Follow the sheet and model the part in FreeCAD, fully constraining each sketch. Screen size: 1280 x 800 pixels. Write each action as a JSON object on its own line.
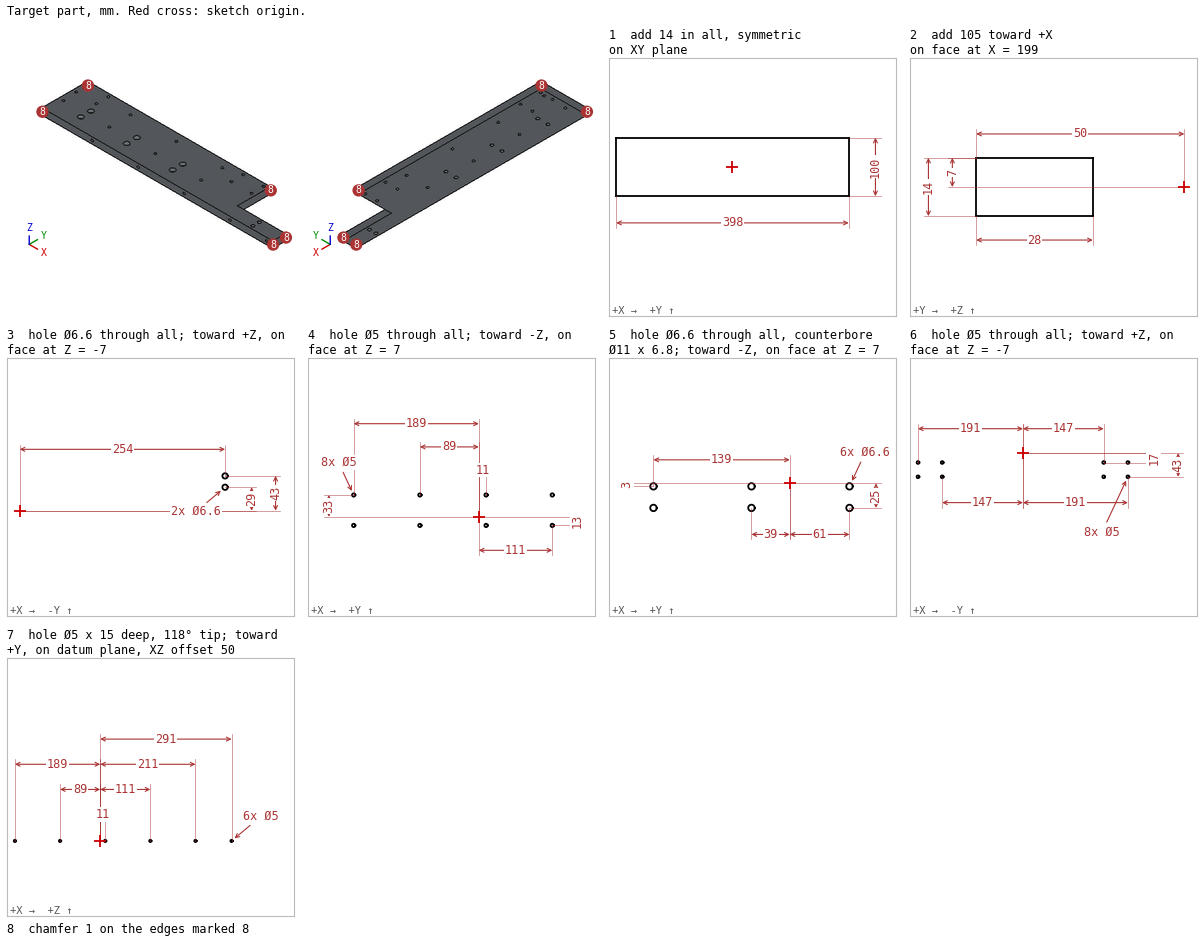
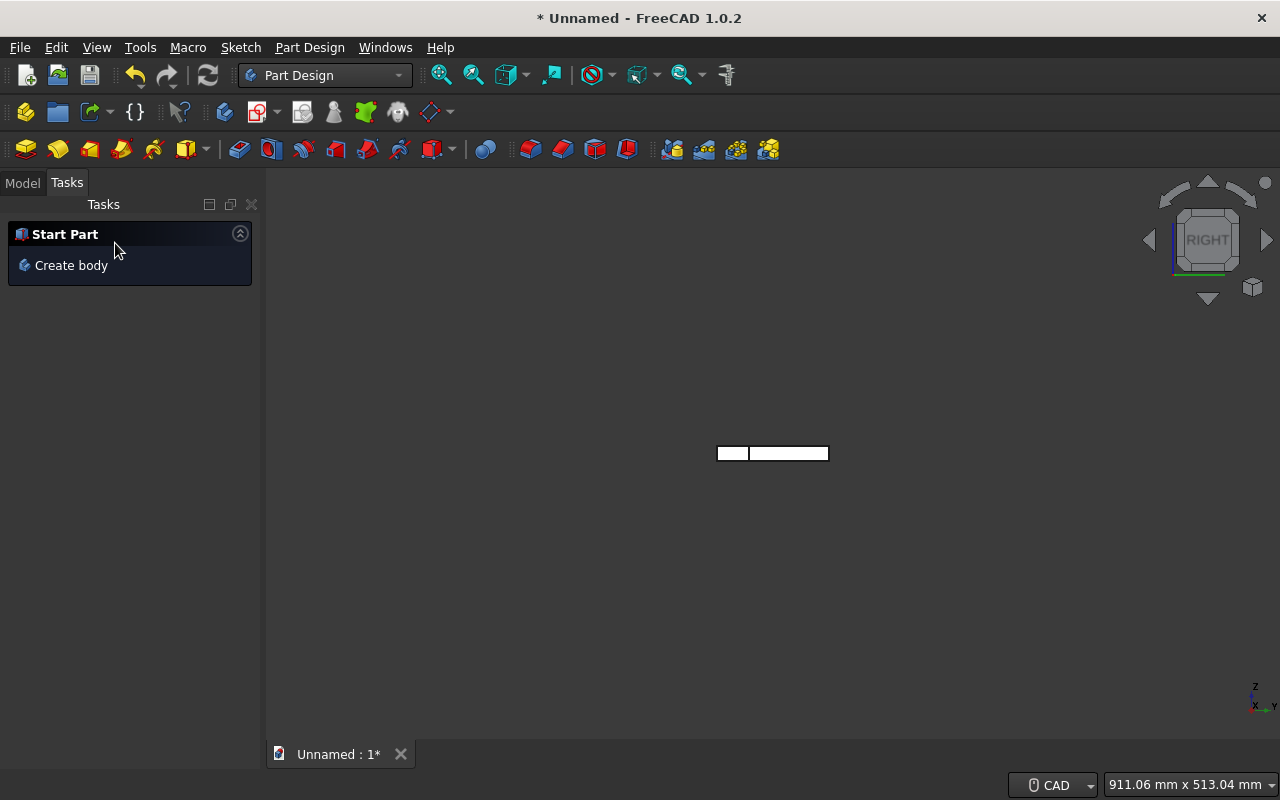
{"action": "key", "text": "5"}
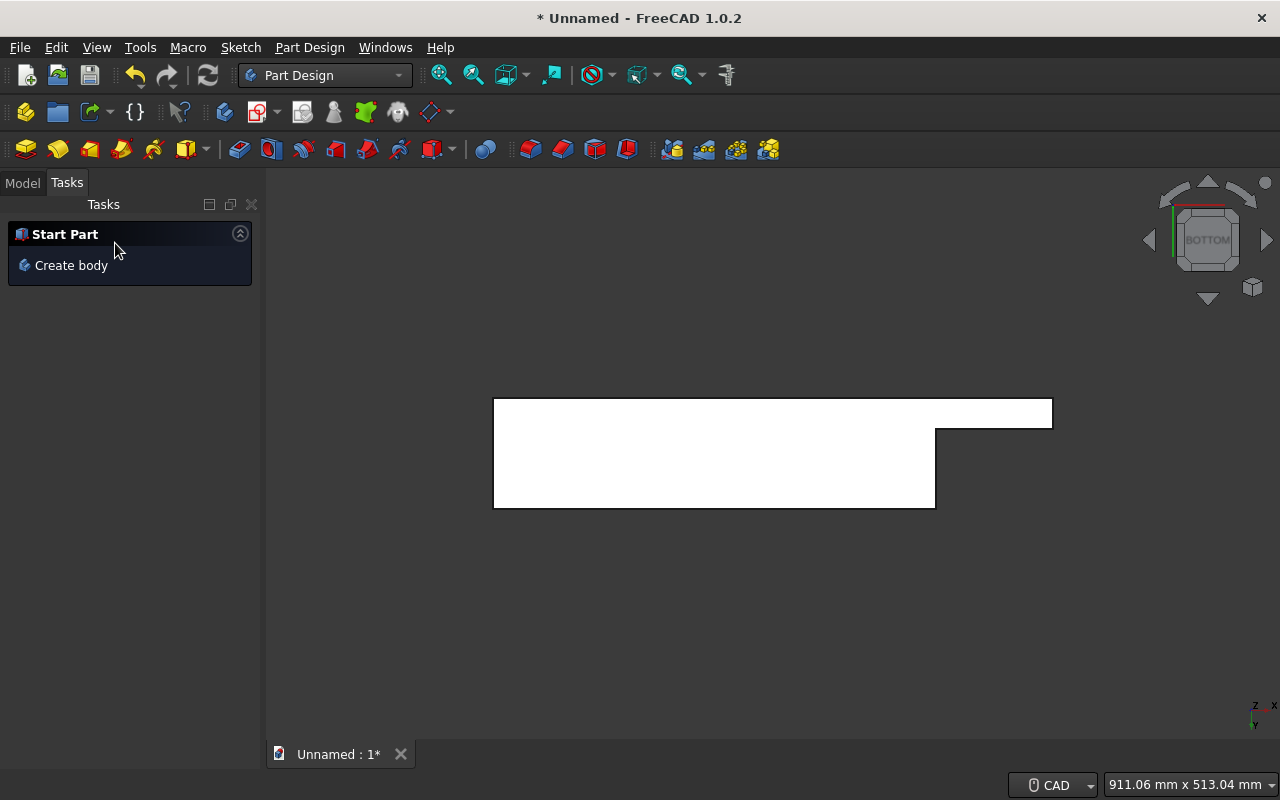
{"action": "left_click", "coordinate": [853, 452]}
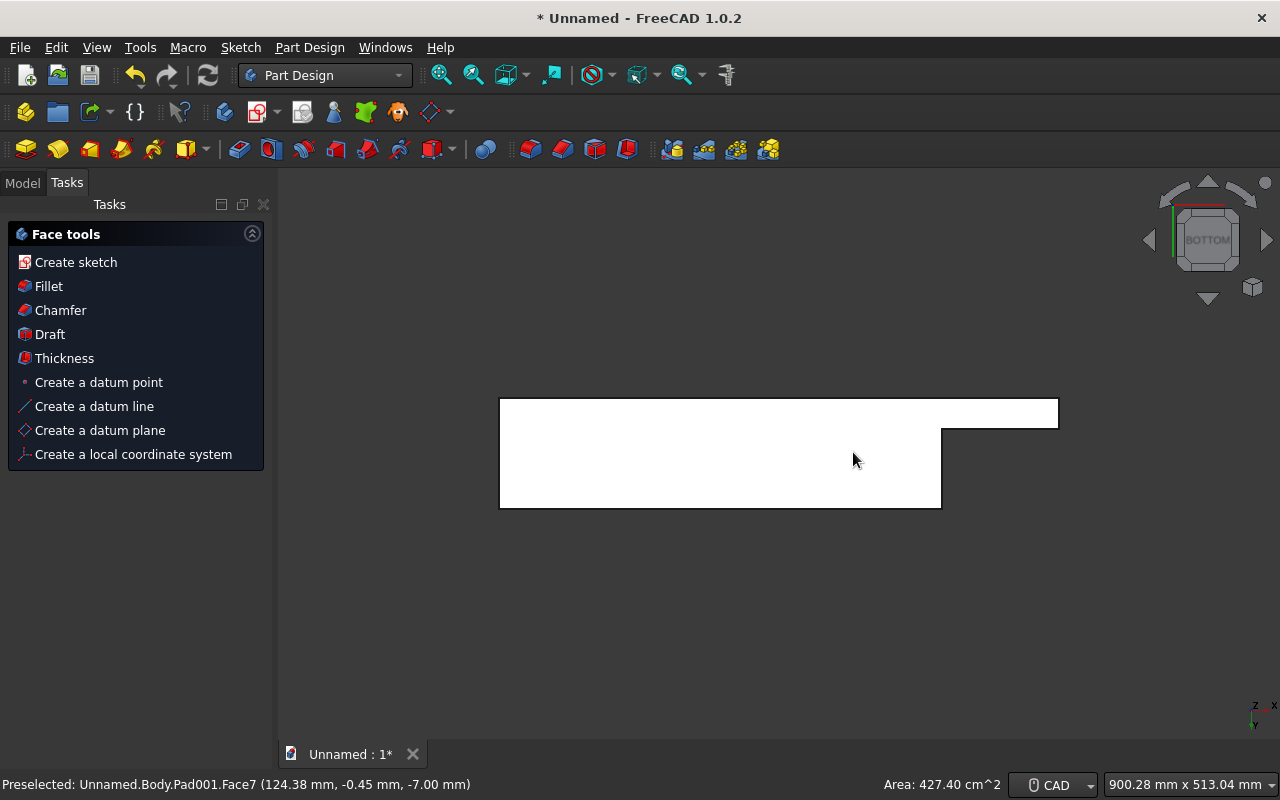
{"action": "left_click", "coordinate": [258, 112]}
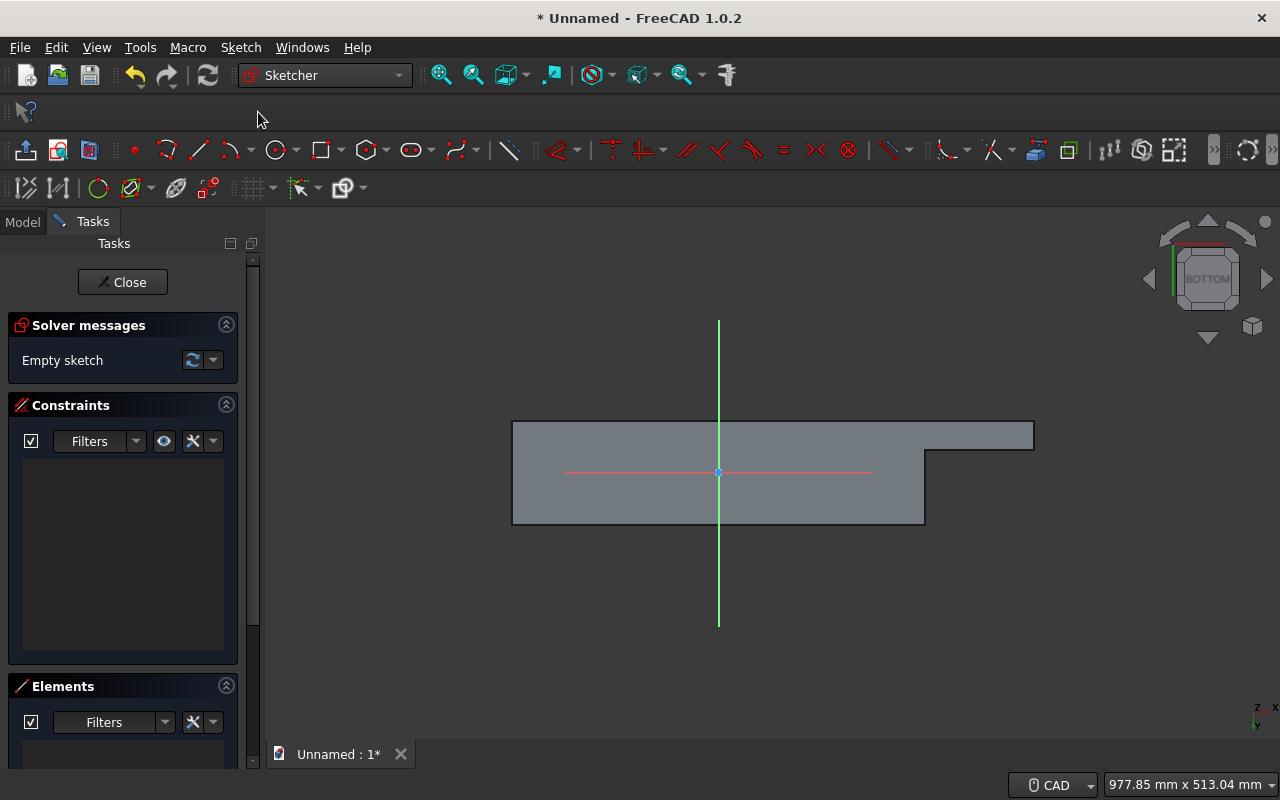
{"action": "scroll", "coordinate": [1000, 433], "scroll_direction": "up", "scroll_amount": 14}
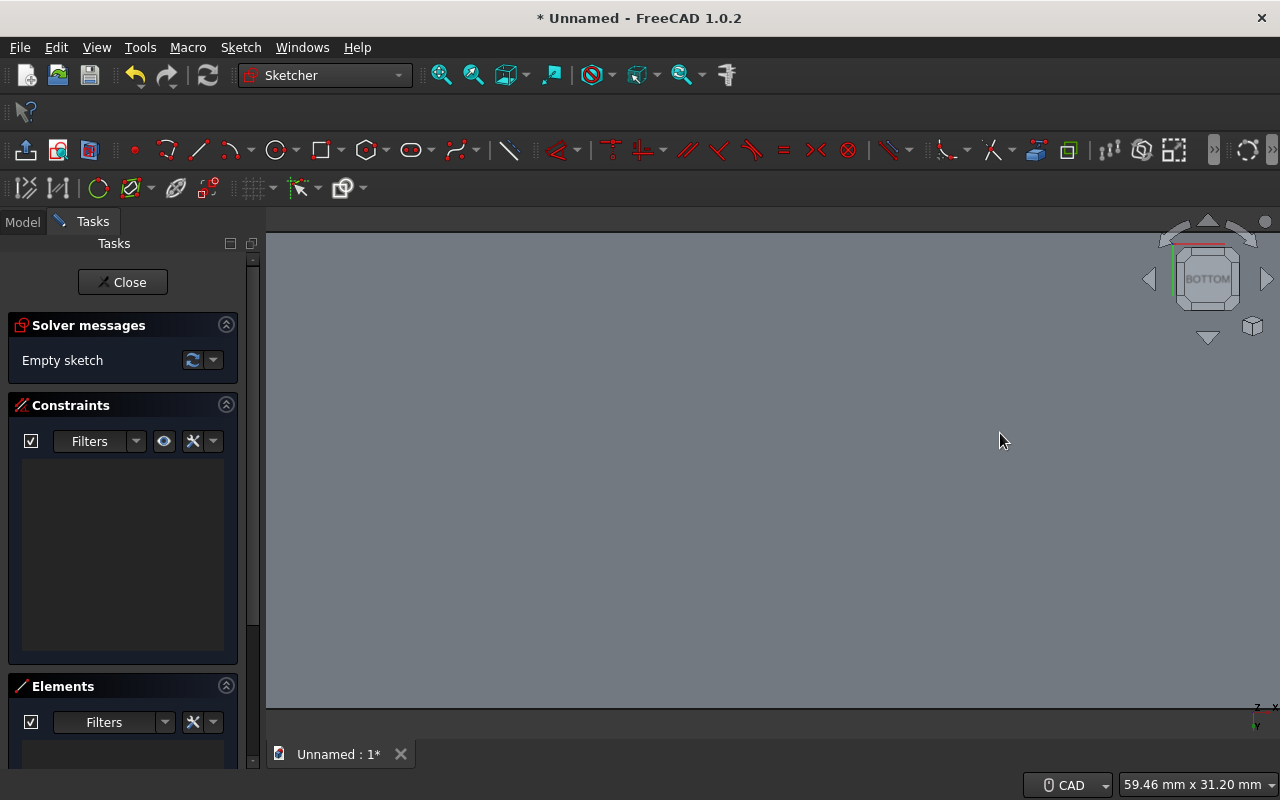
{"action": "key", "text": "g c"}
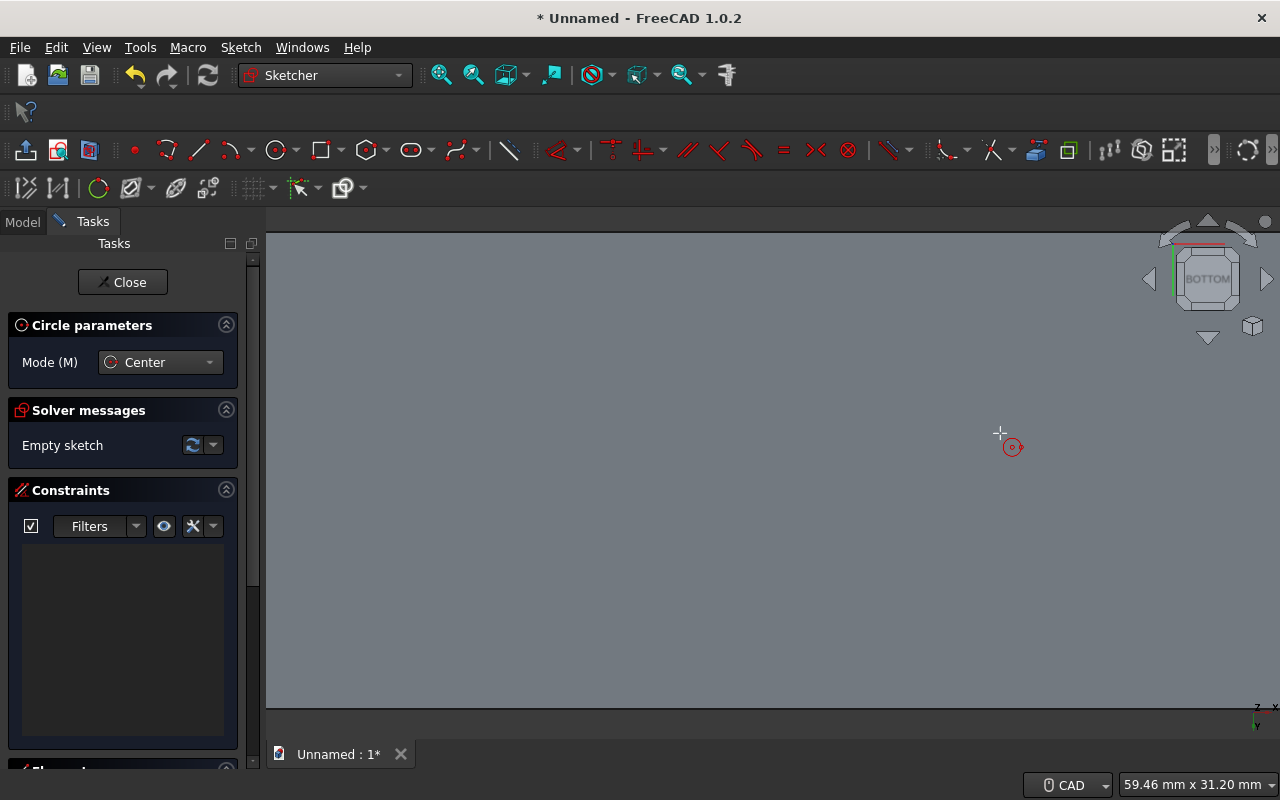
{"action": "left_click", "coordinate": [692, 351]}
{"action": "left_click", "coordinate": [732, 311]}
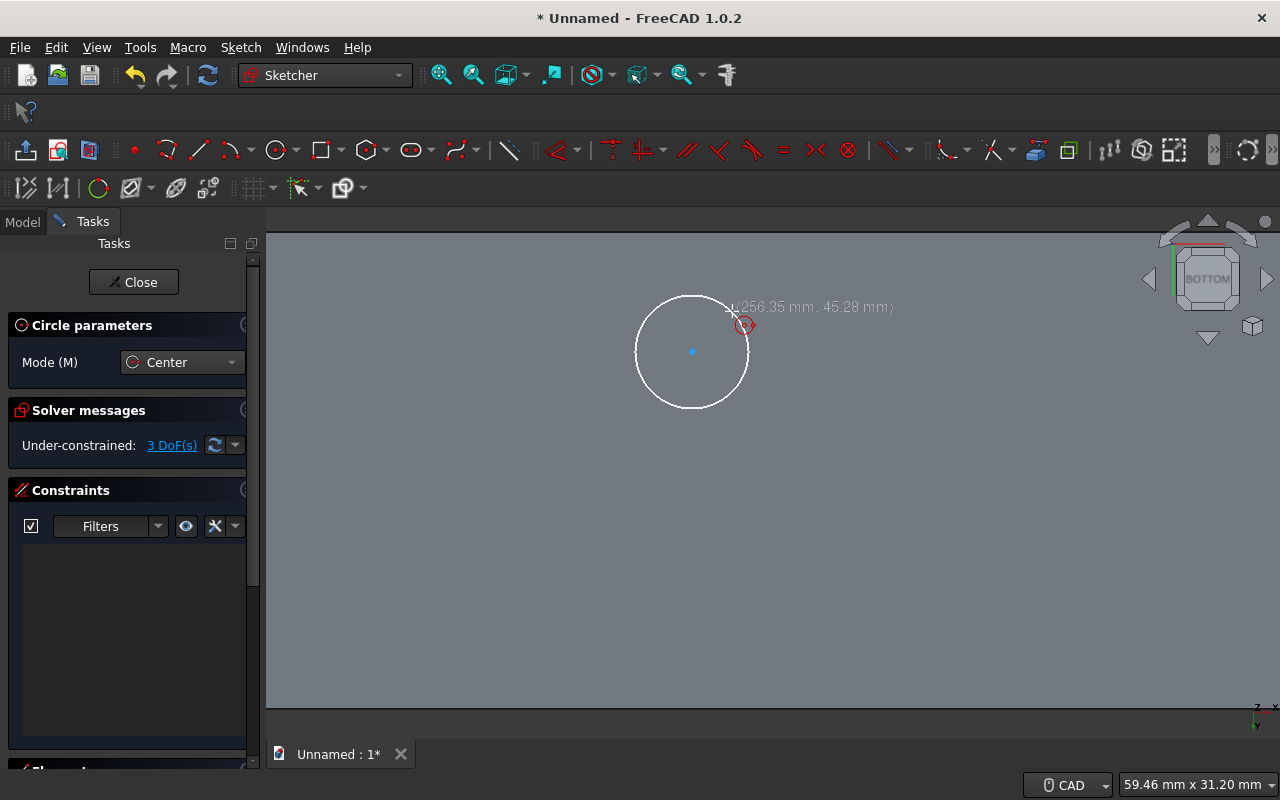
{"action": "left_click", "coordinate": [692, 590]}
{"action": "left_click", "coordinate": [732, 550]}
{"action": "key", "text": "Escape"}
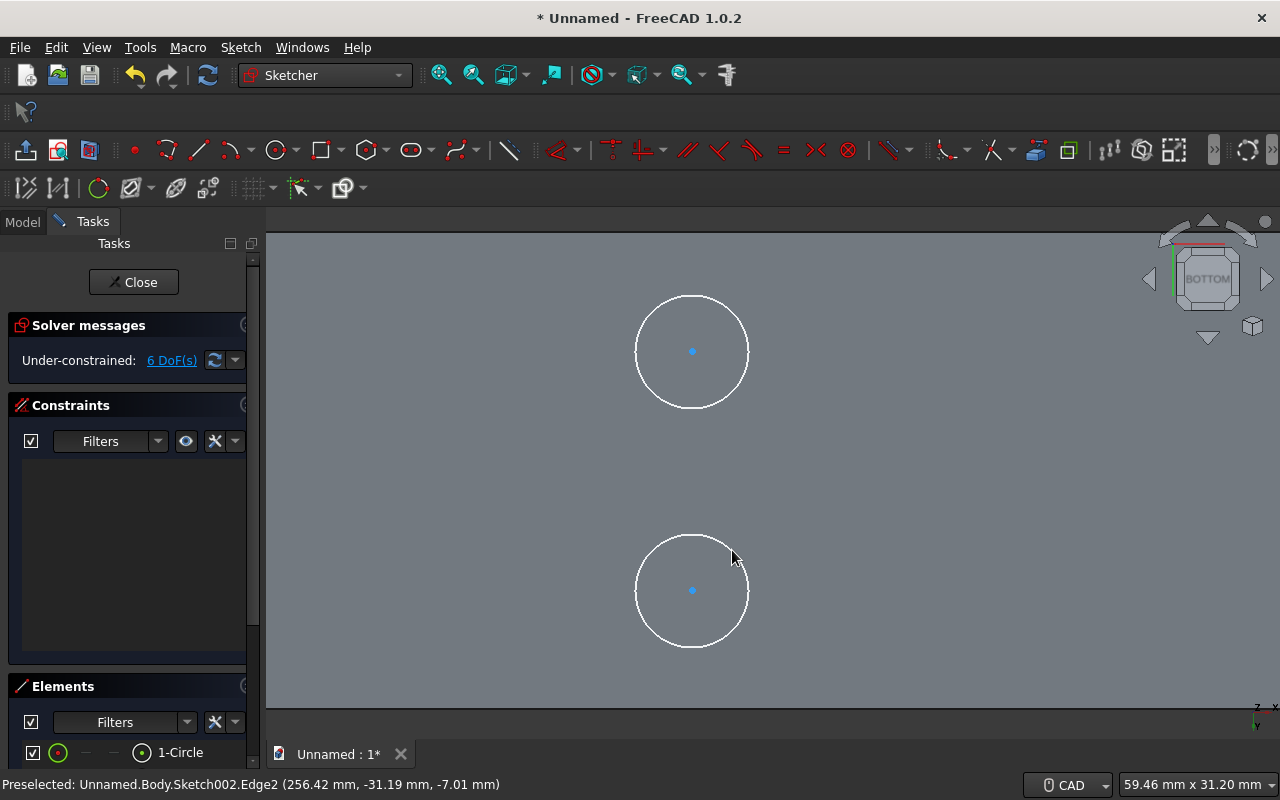
{"action": "left_click", "coordinate": [732, 312]}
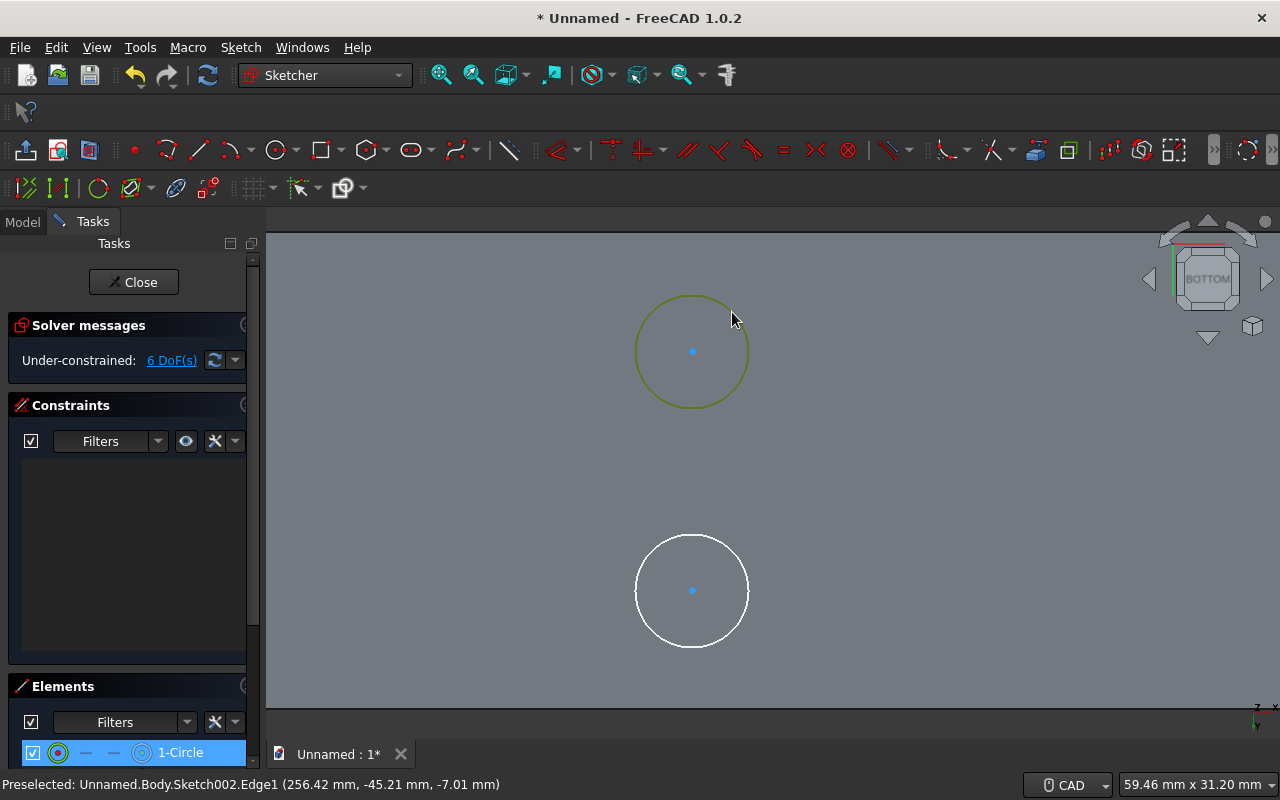
{"action": "left_click", "coordinate": [732, 551]}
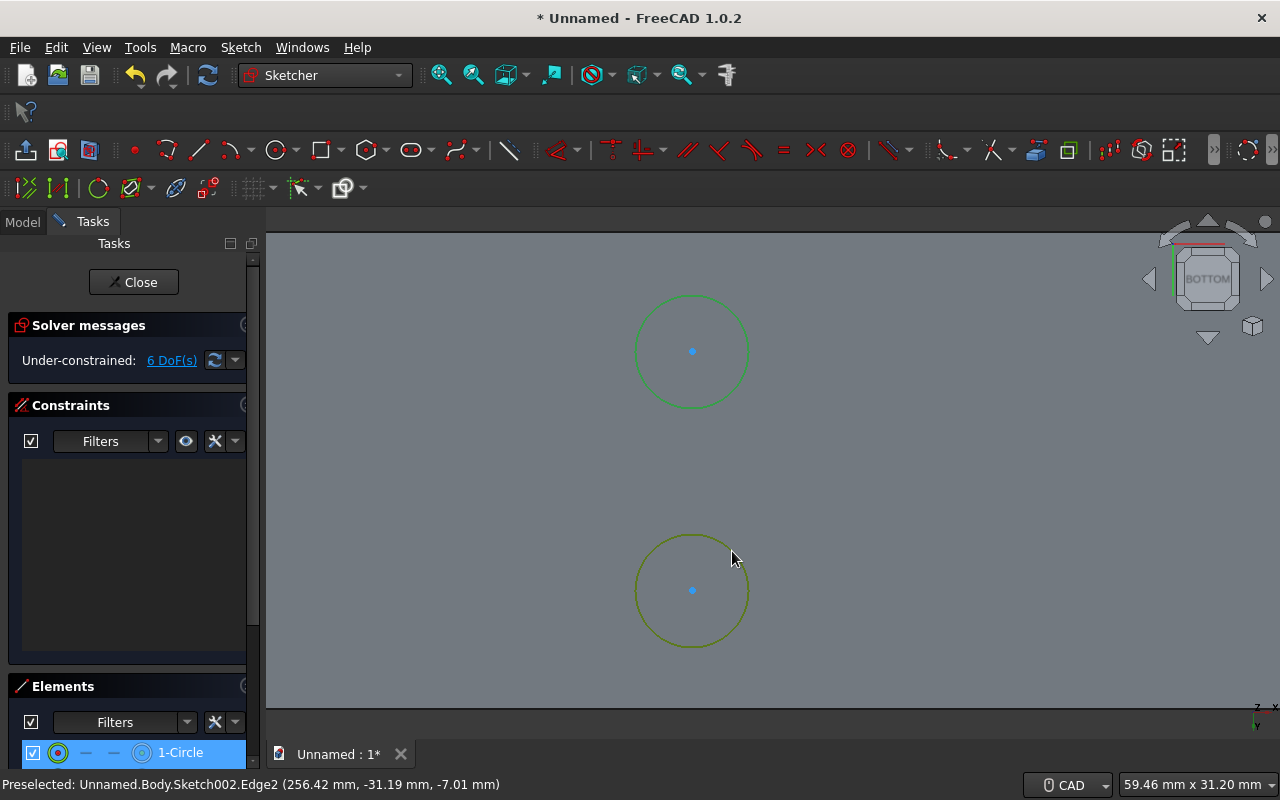
{"action": "key", "text": "e"}